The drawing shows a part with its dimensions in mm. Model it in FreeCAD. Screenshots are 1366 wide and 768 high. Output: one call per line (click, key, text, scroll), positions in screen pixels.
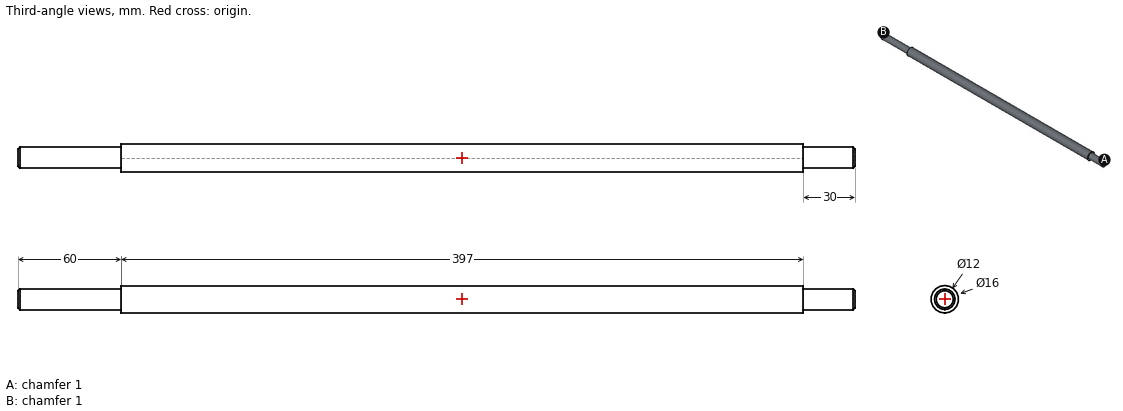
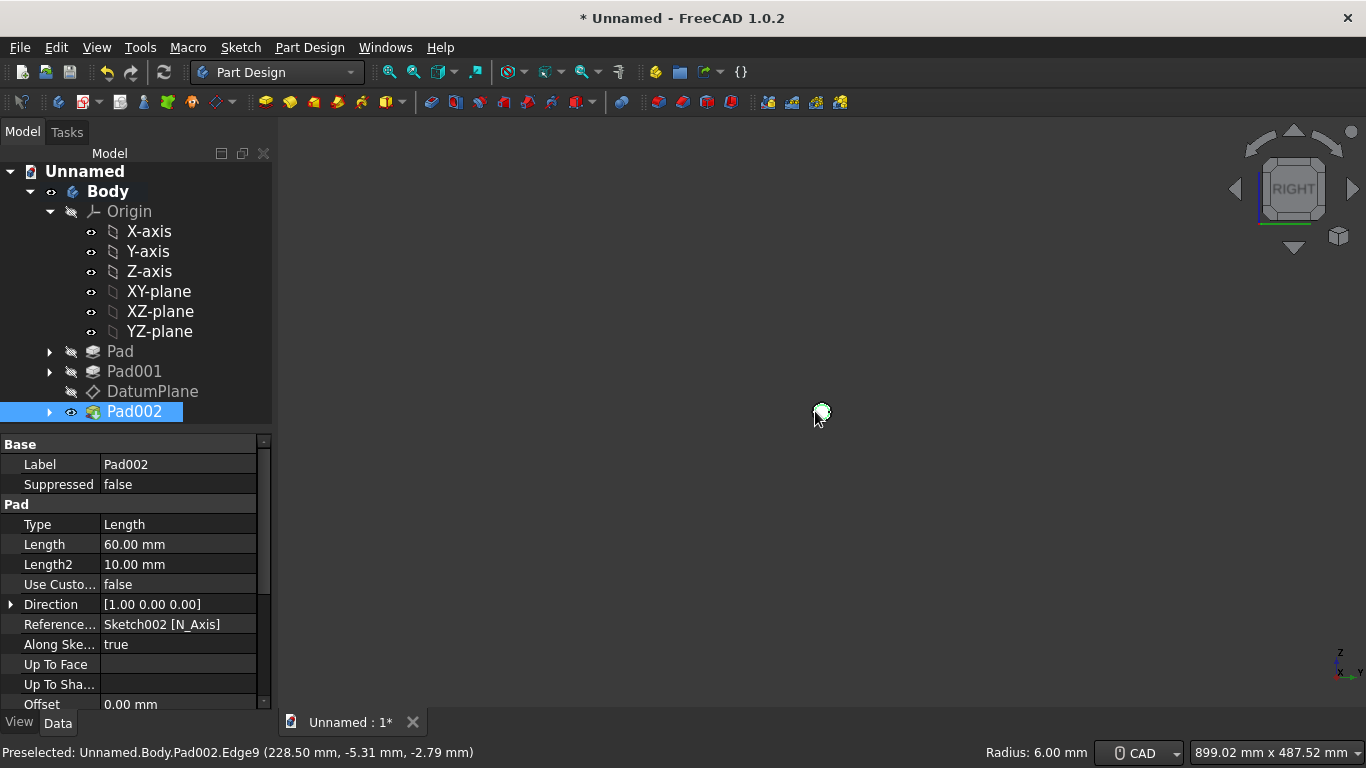
click(684, 102)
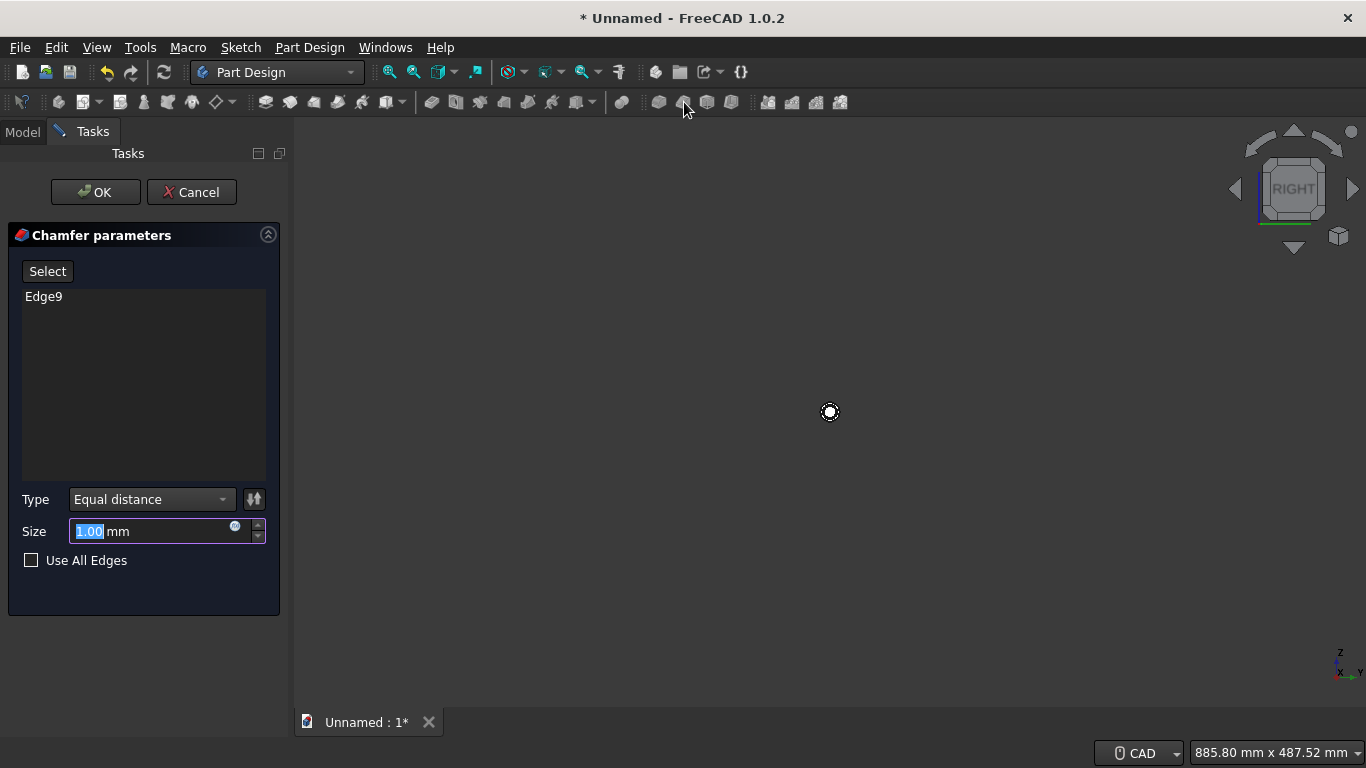
text(1)
key(Tab)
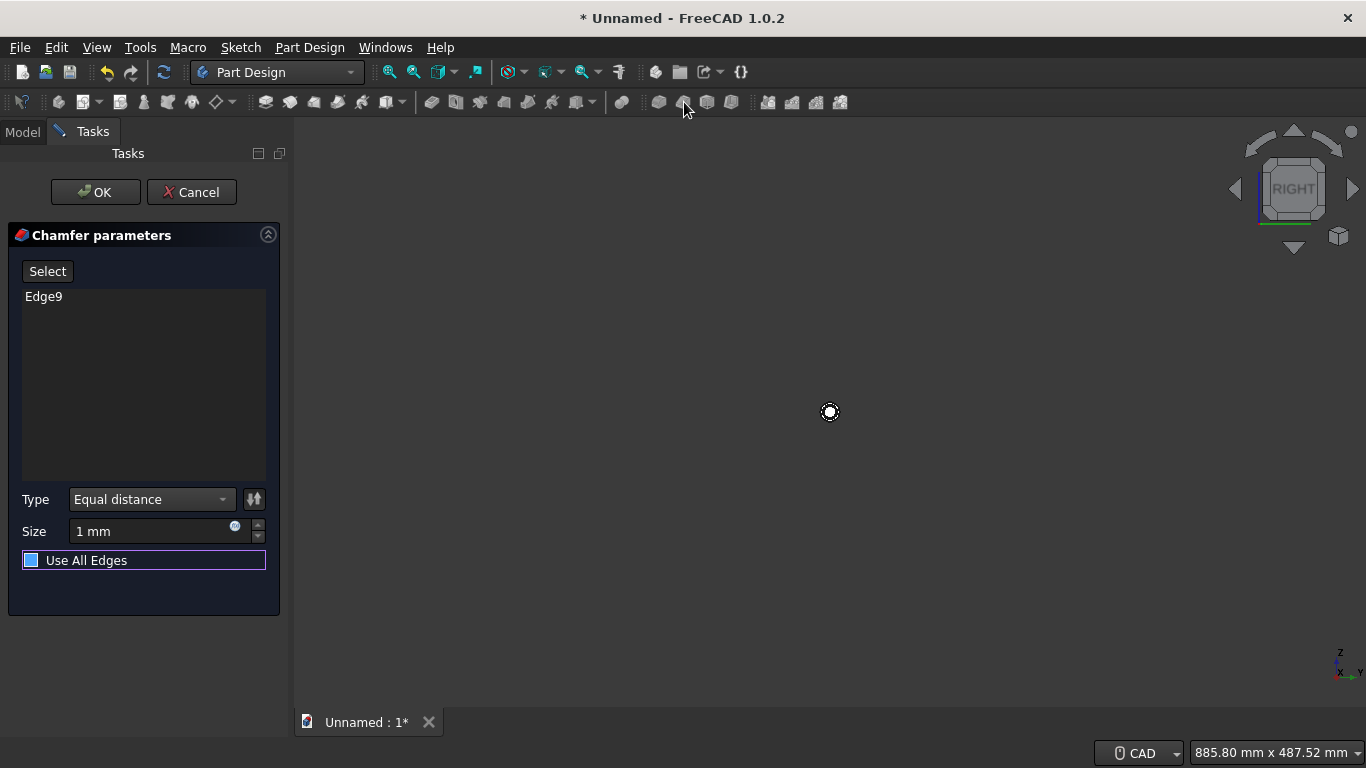
click(96, 192)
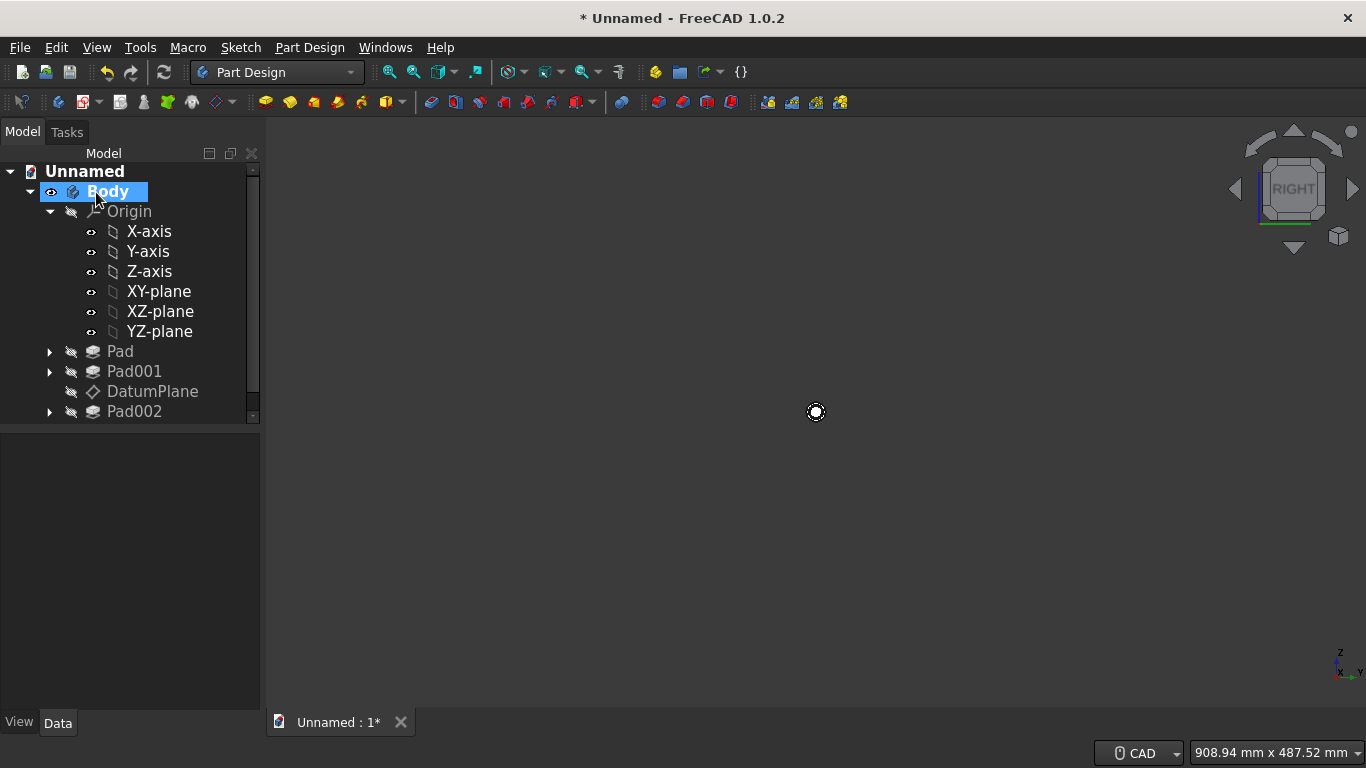
click(390, 72)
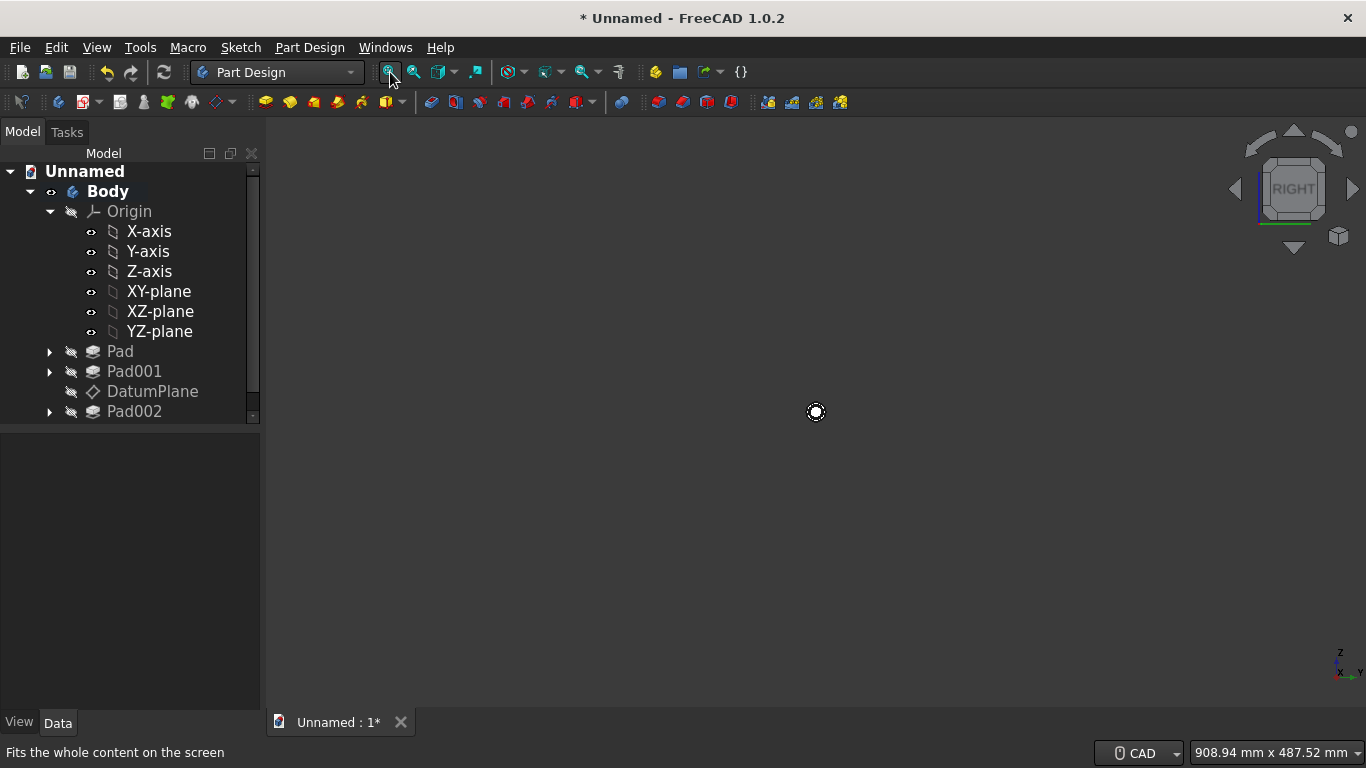
key(0)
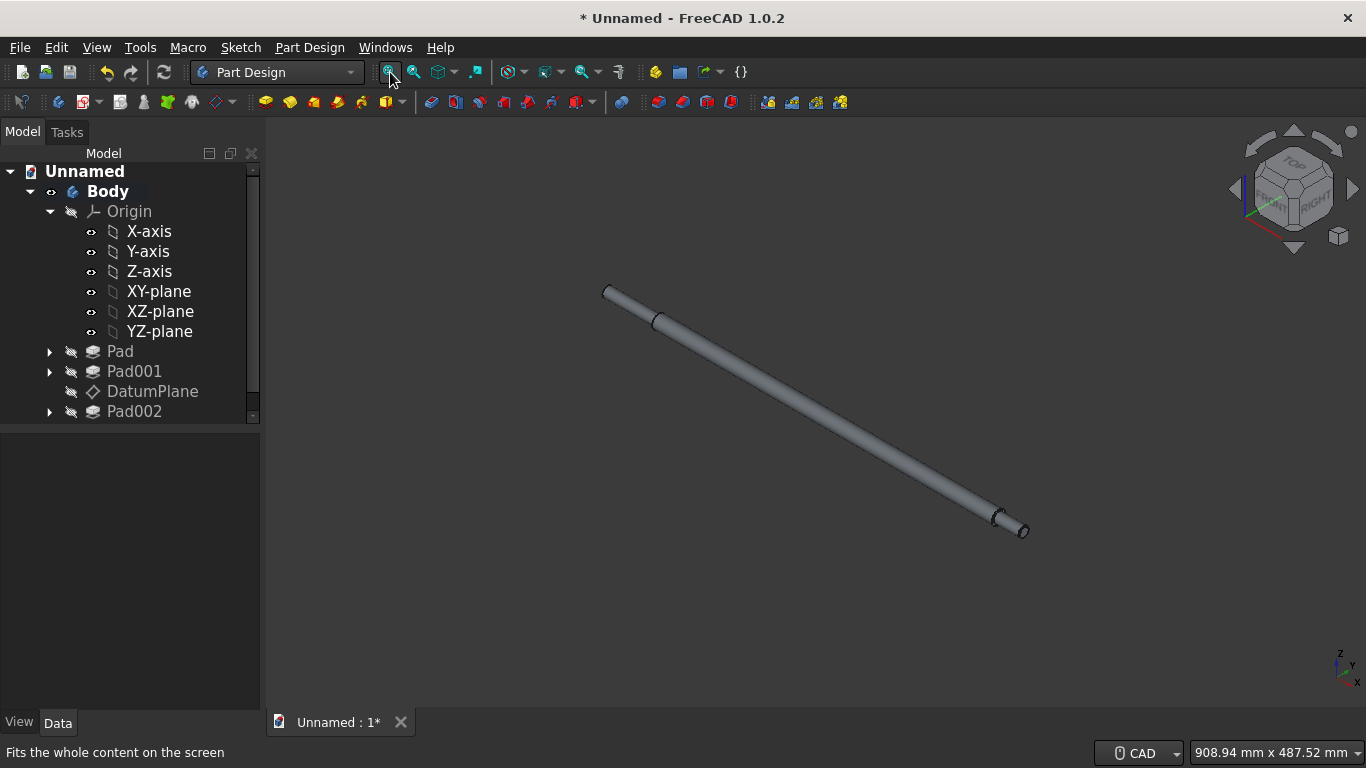
key(v)
key(f)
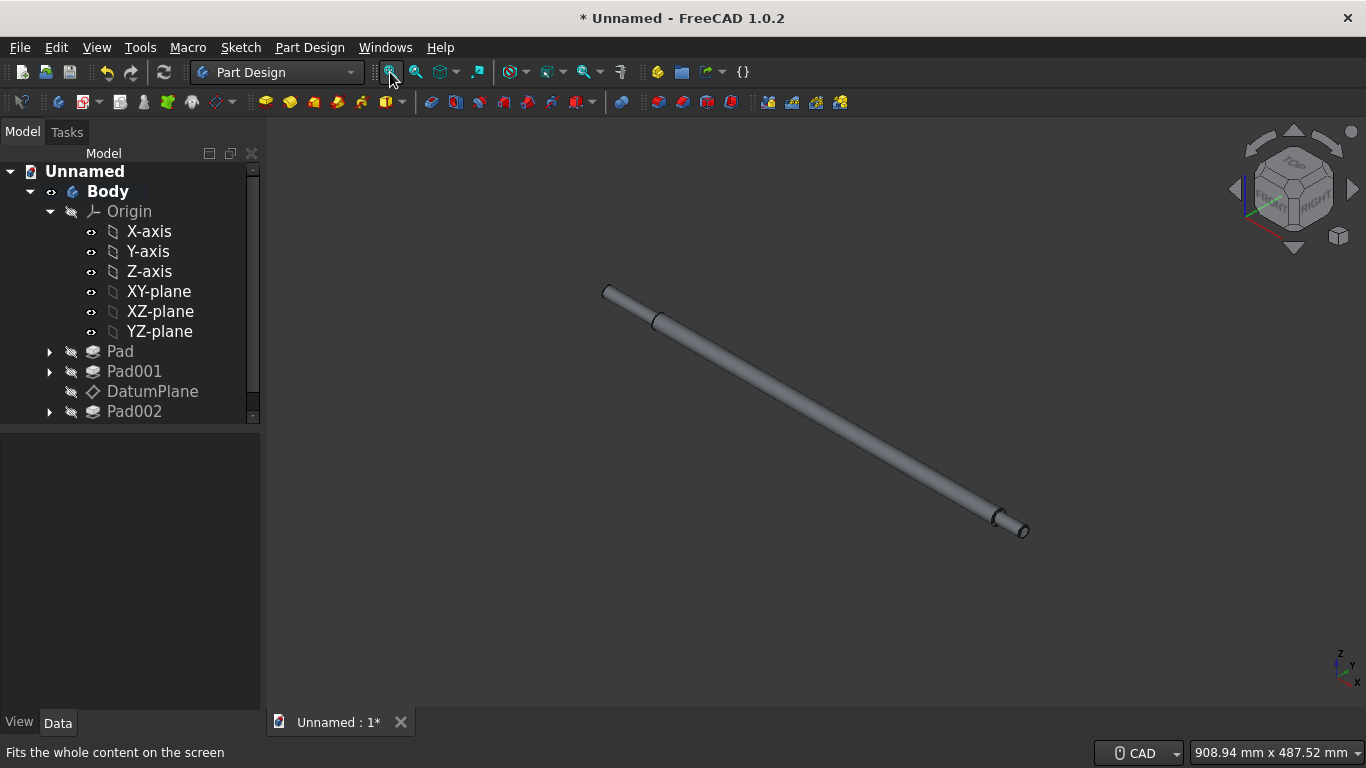
click(602, 294)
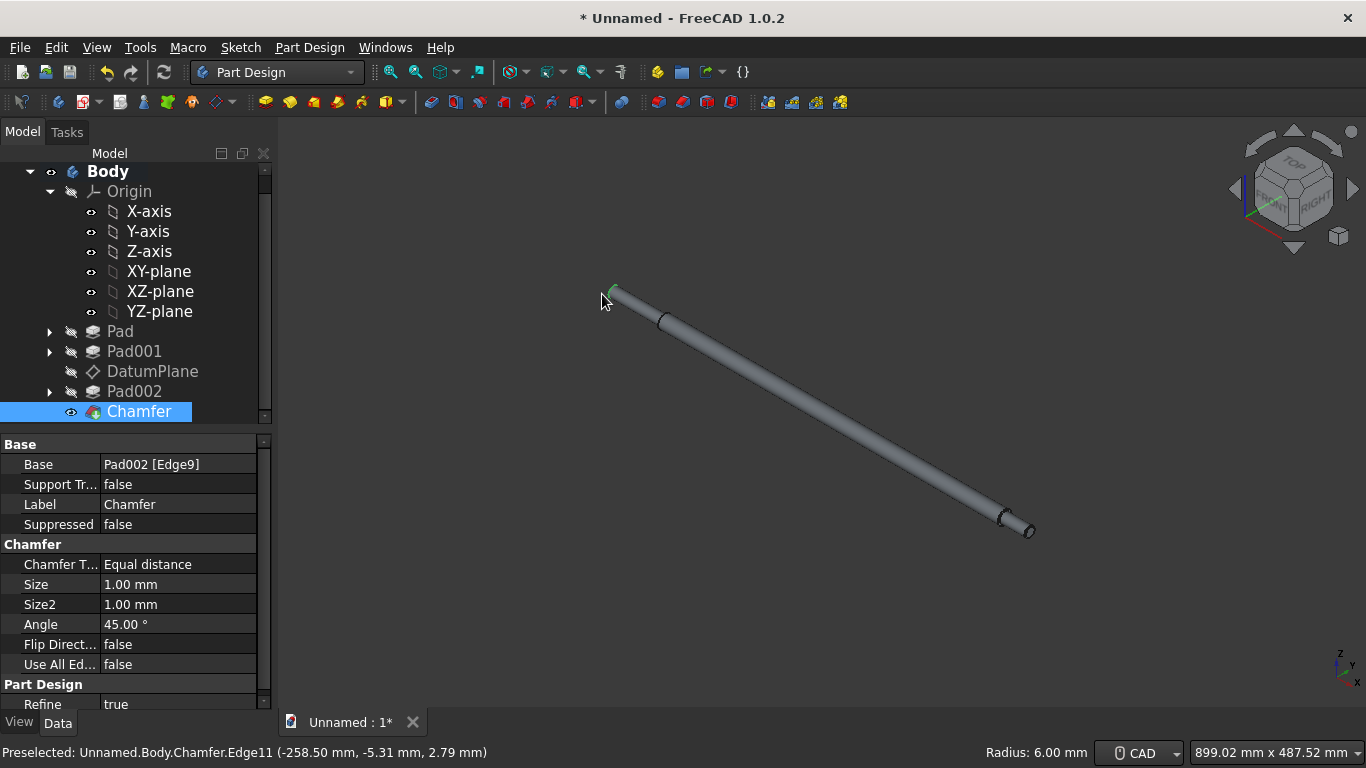
click(684, 102)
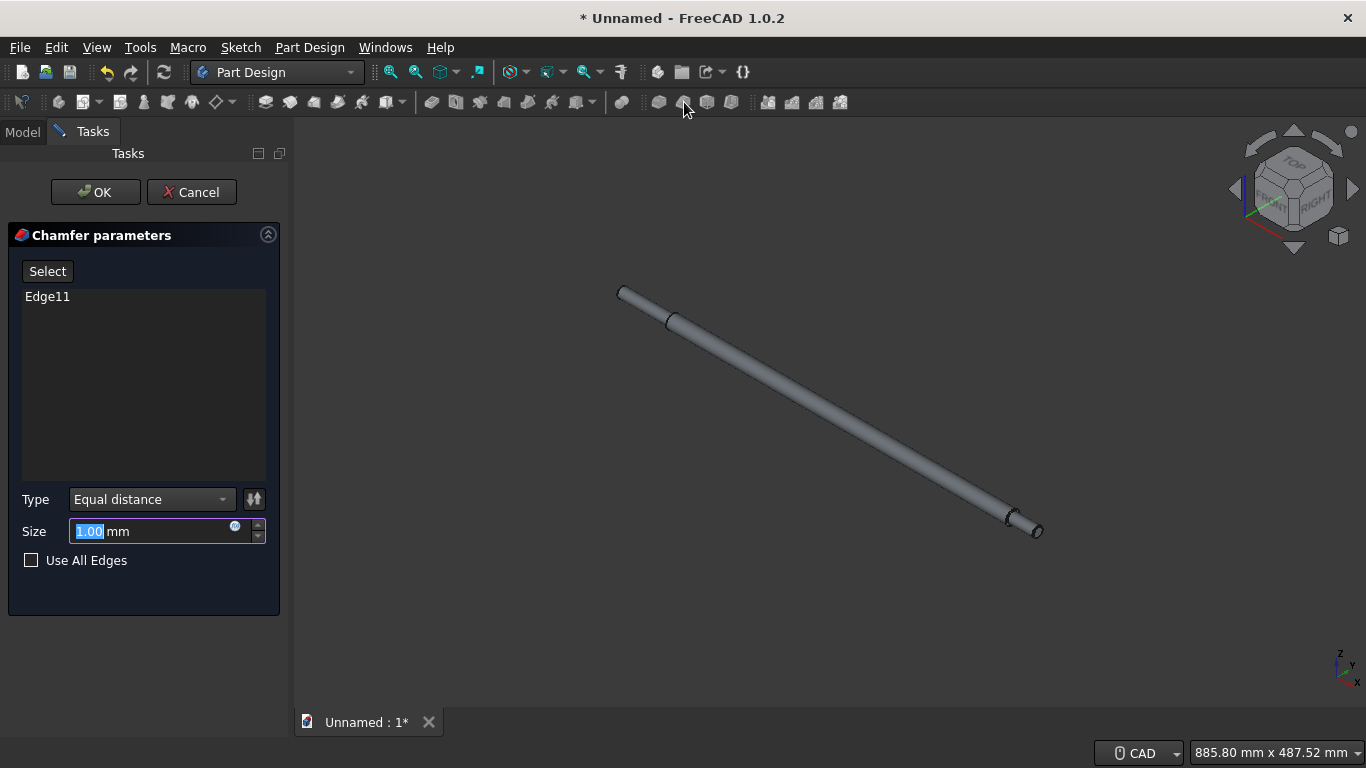
text(1)
key(Tab)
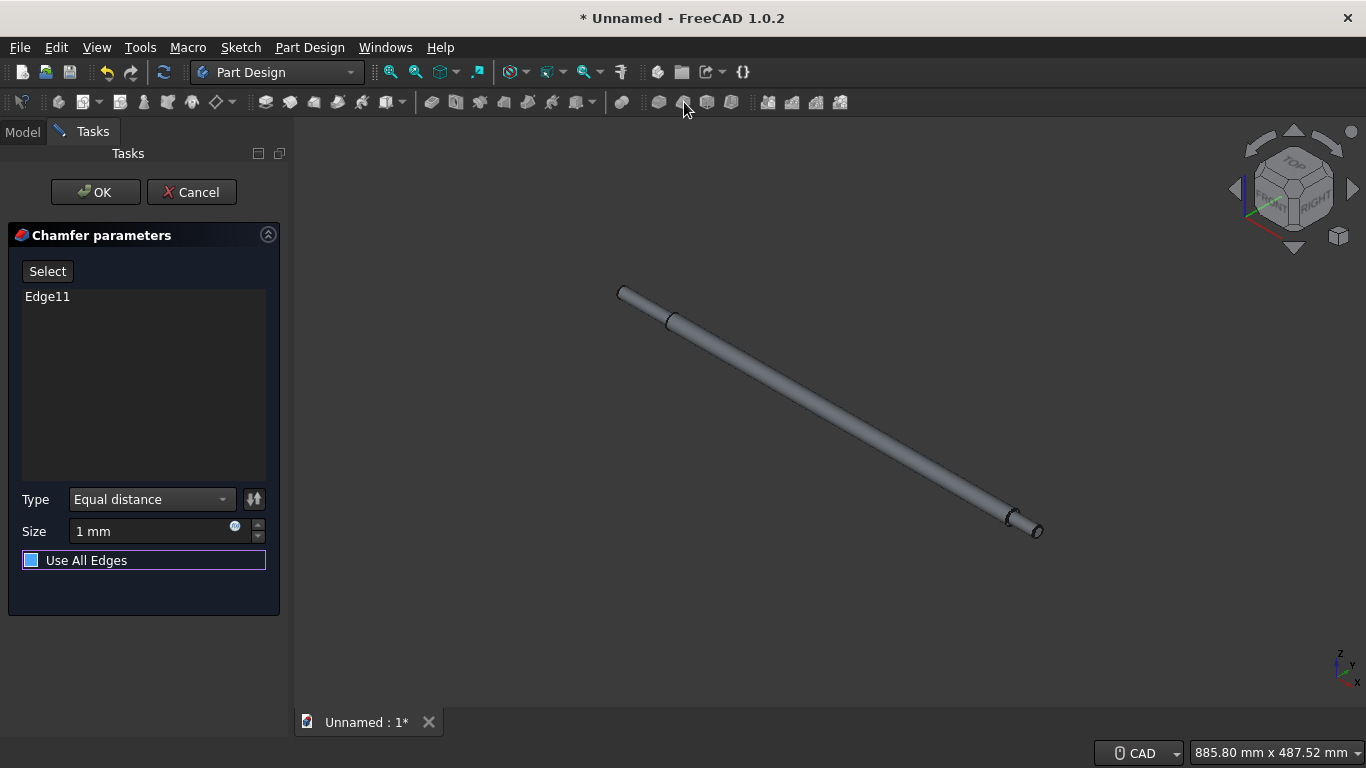
click(96, 192)